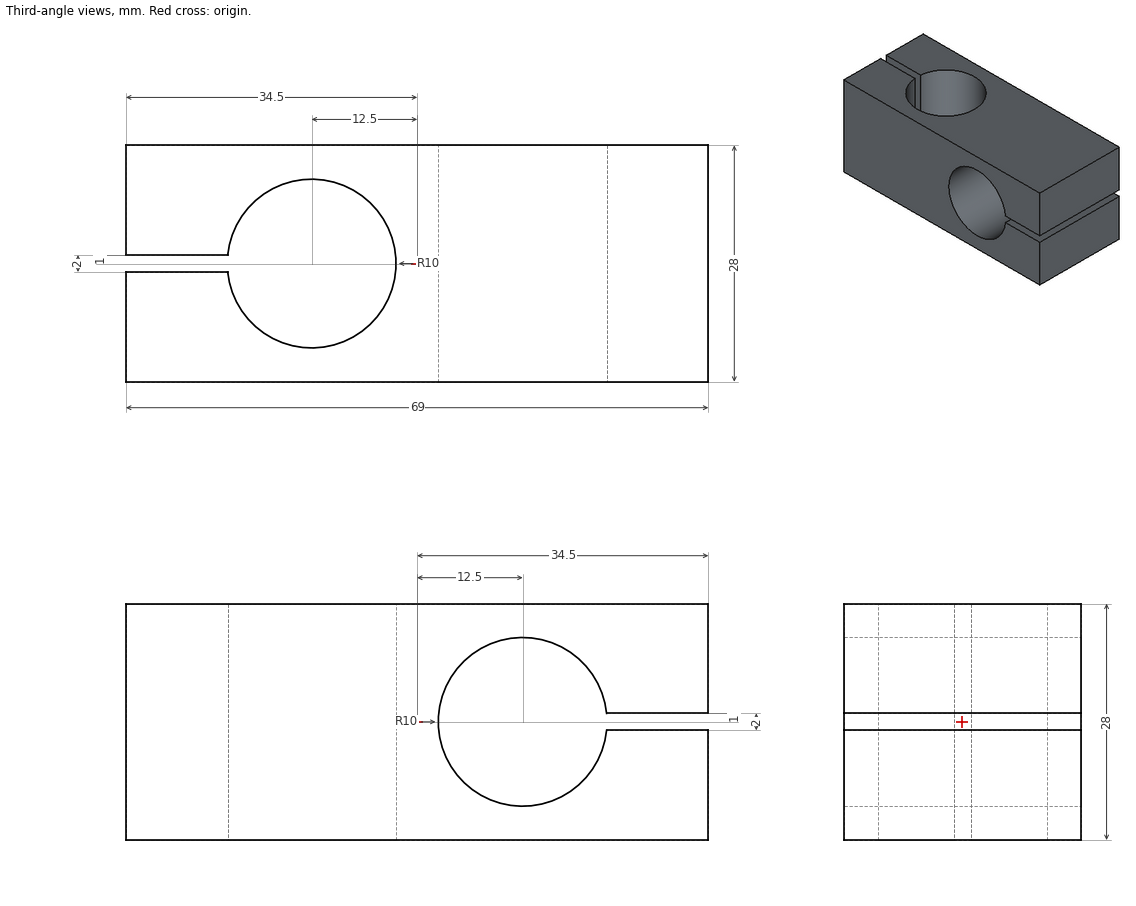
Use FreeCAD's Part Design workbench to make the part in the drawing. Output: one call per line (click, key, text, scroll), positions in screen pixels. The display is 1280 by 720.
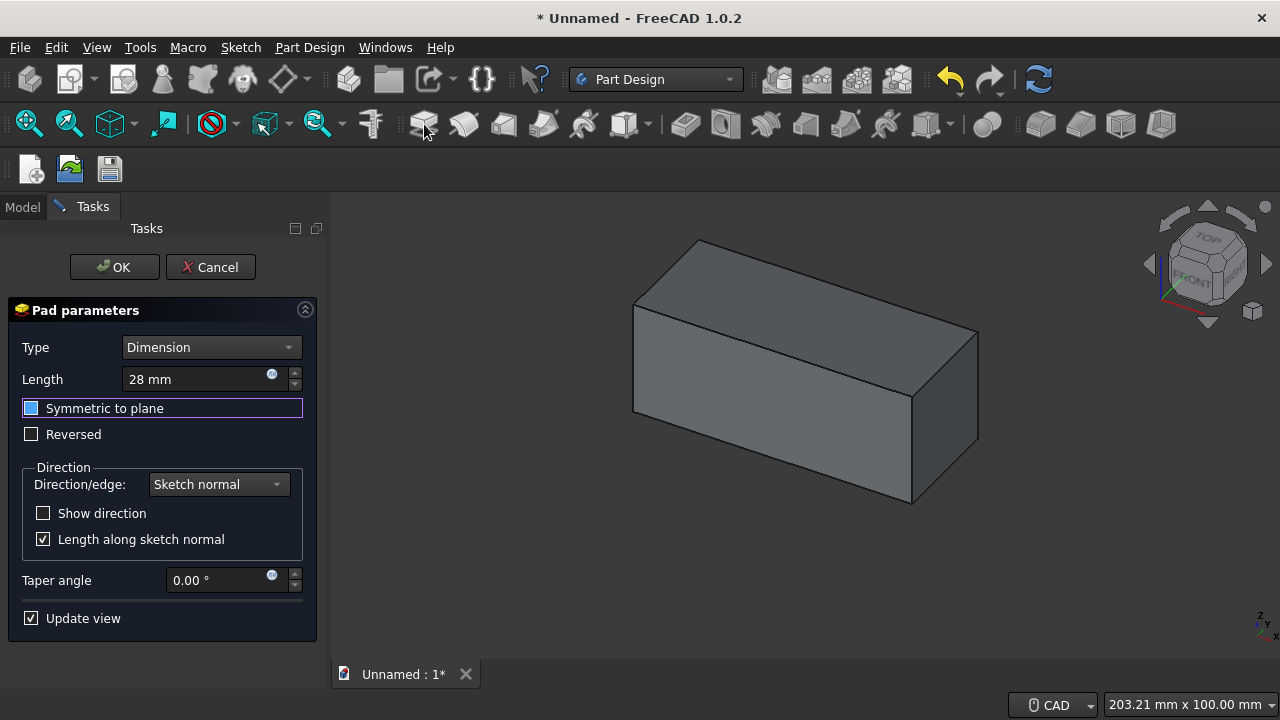
click(30, 408)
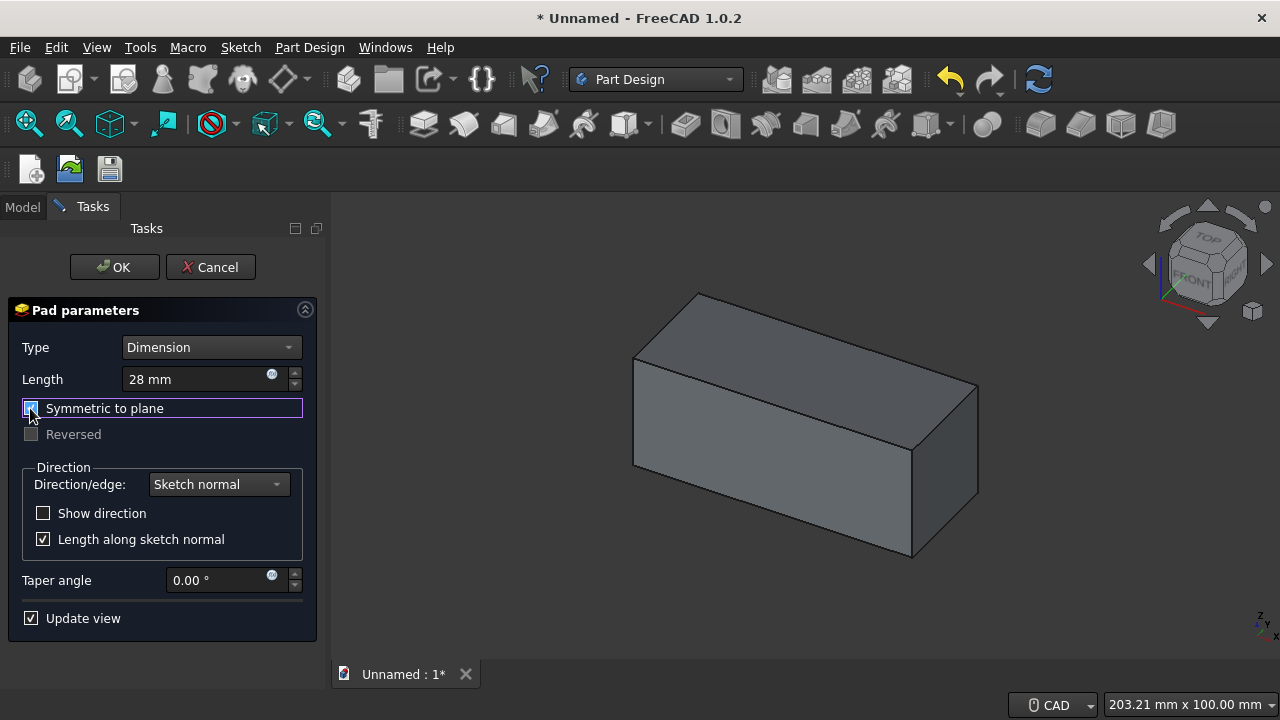
click(115, 267)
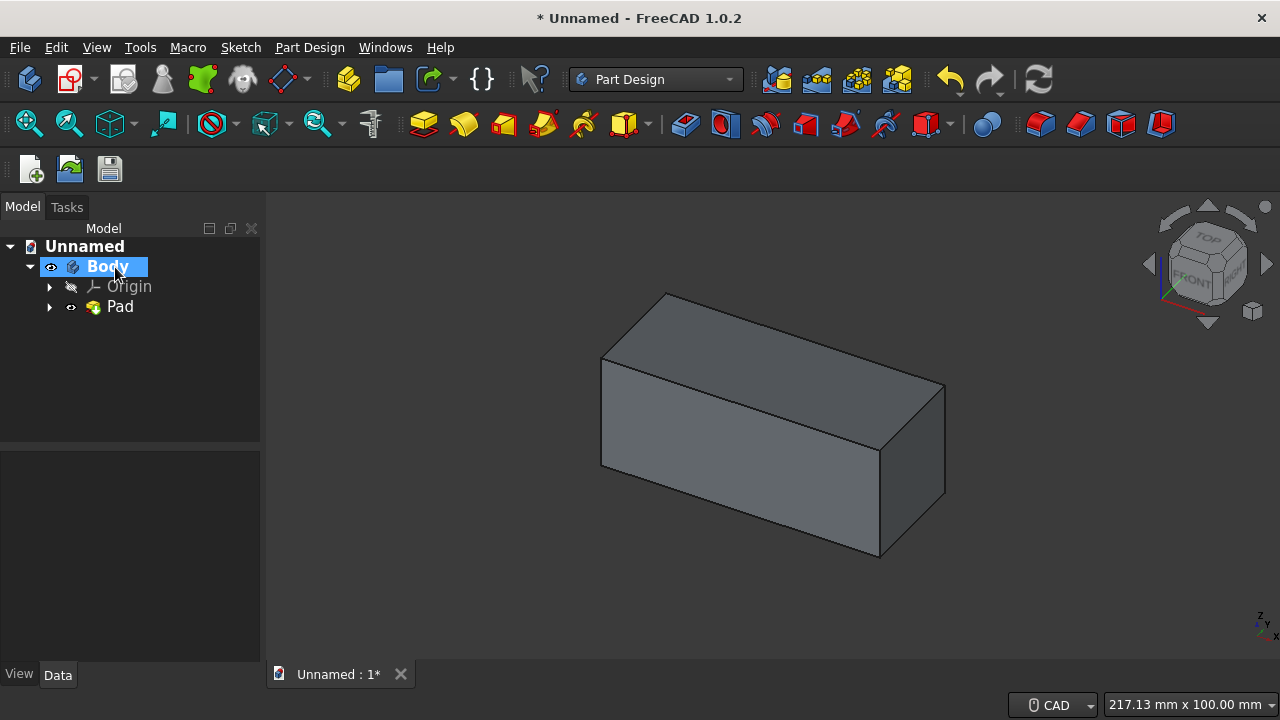
click(853, 397)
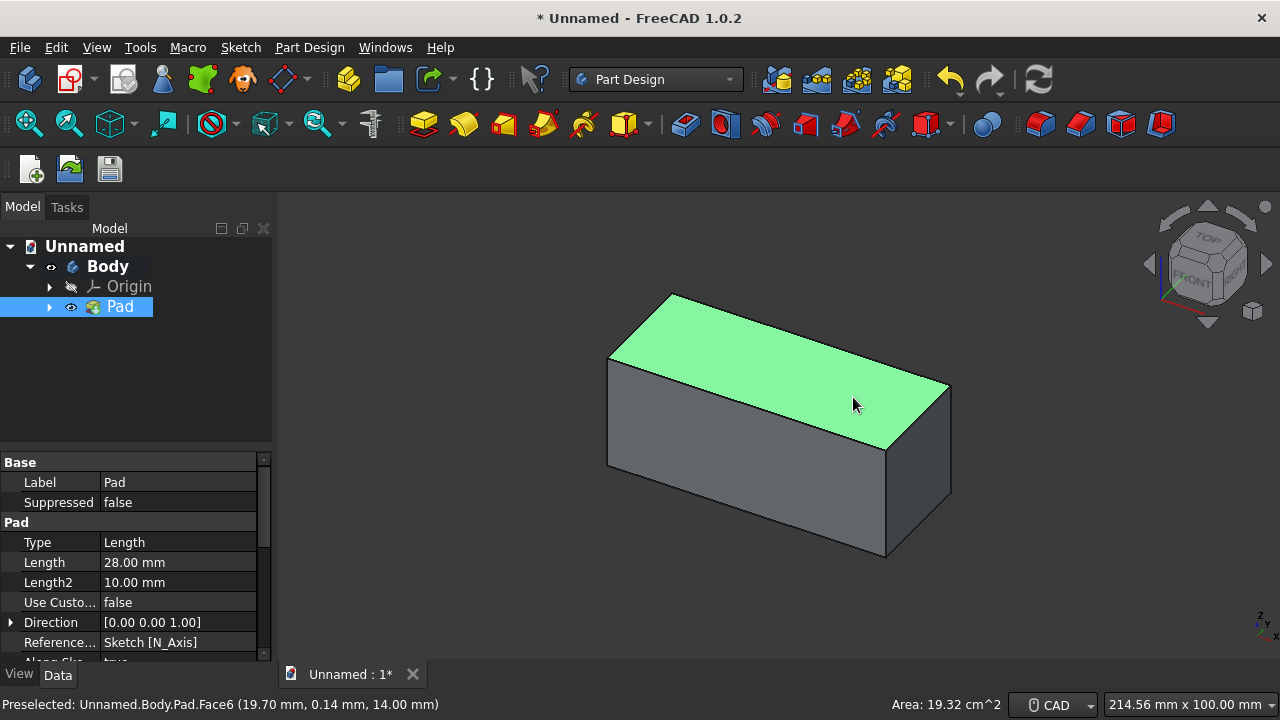
click(70, 80)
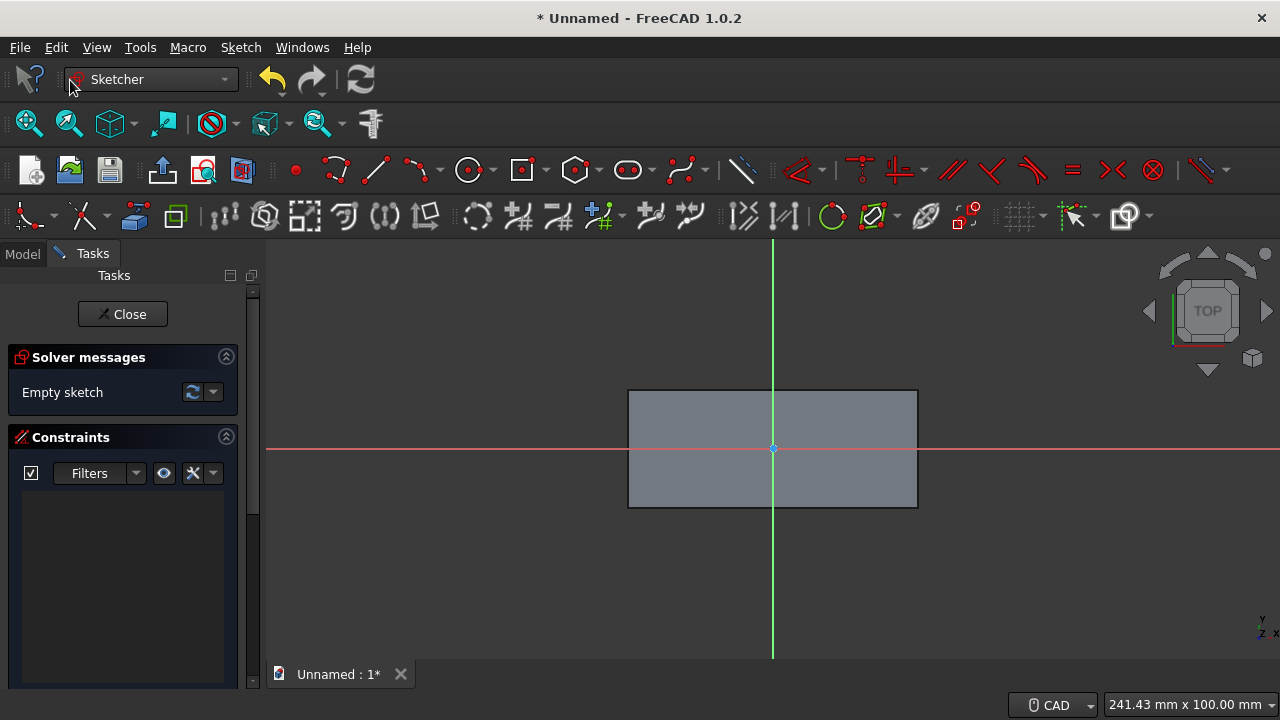
scroll(699, 449, up, 7)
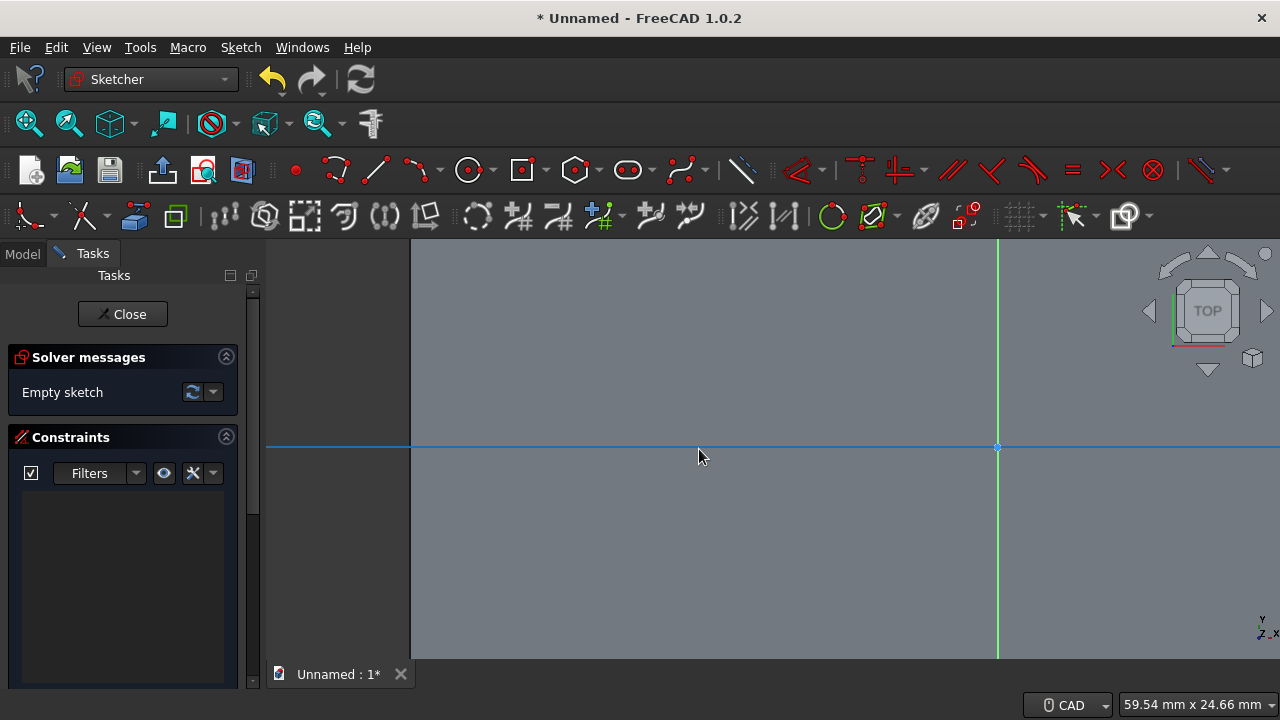
click(336, 170)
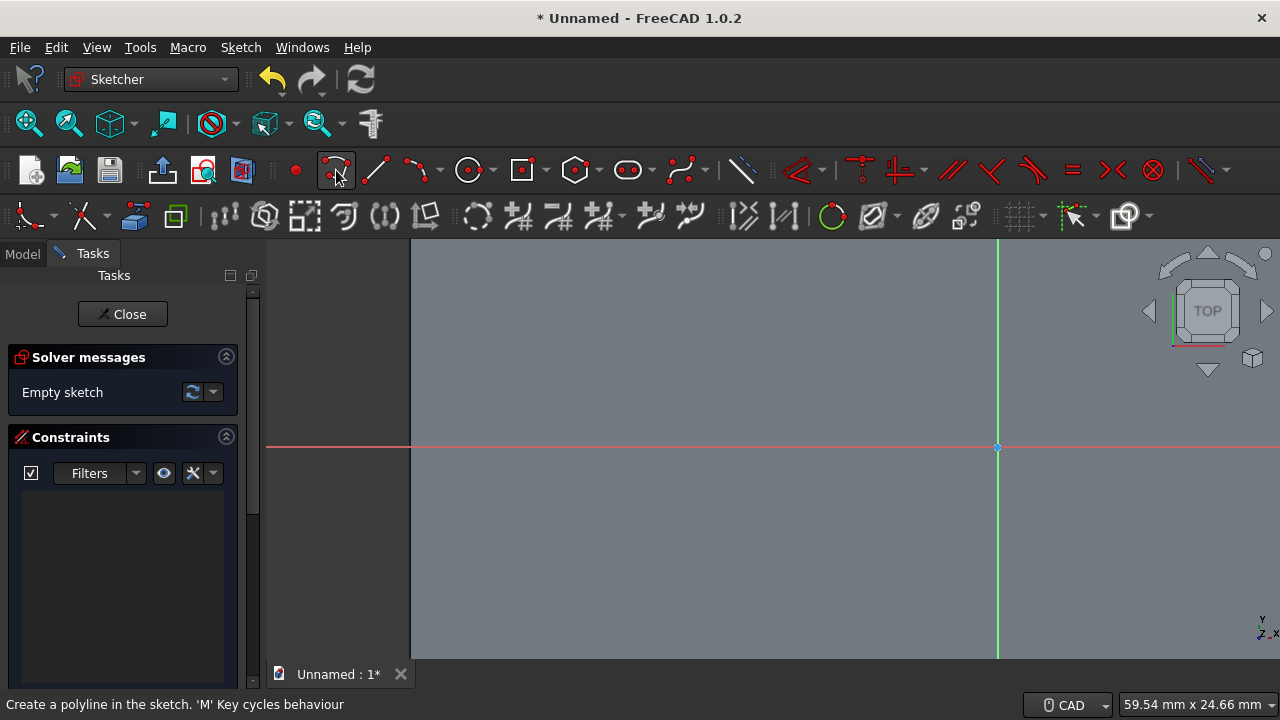
click(615, 430)
click(410, 430)
click(410, 465)
click(615, 465)
right_click(615, 465)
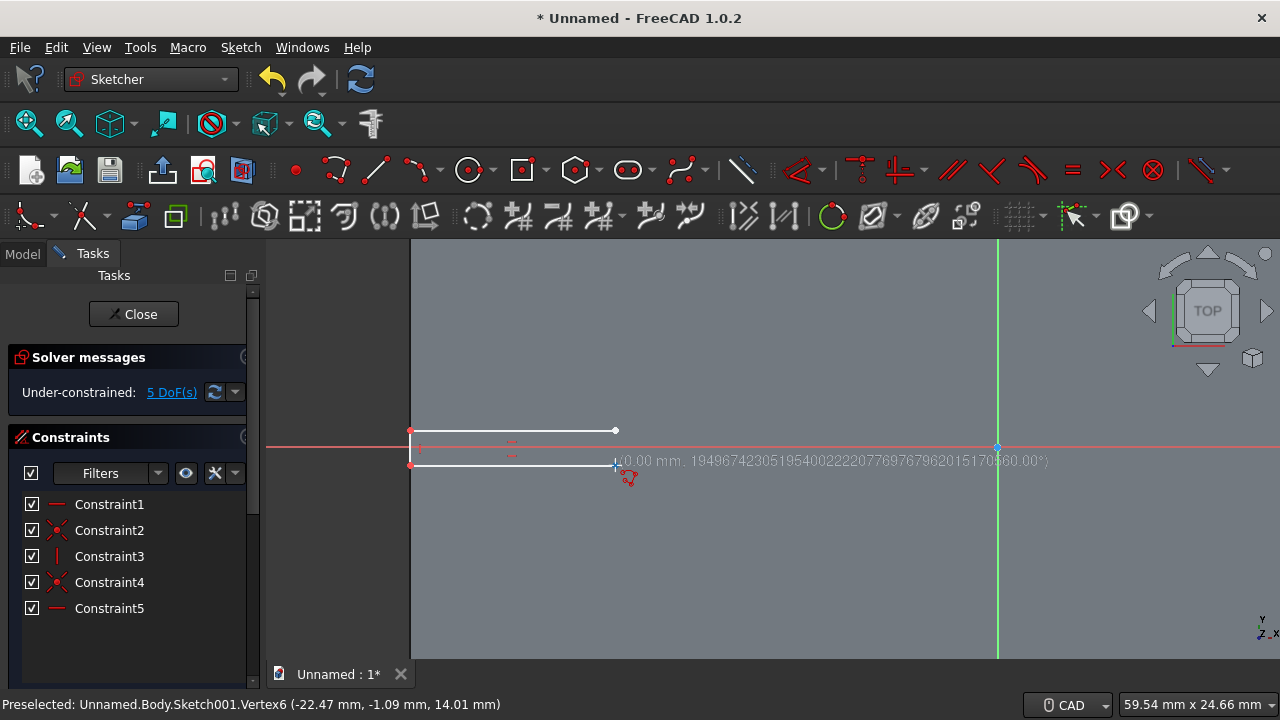
key(g)
key(3)
key(a)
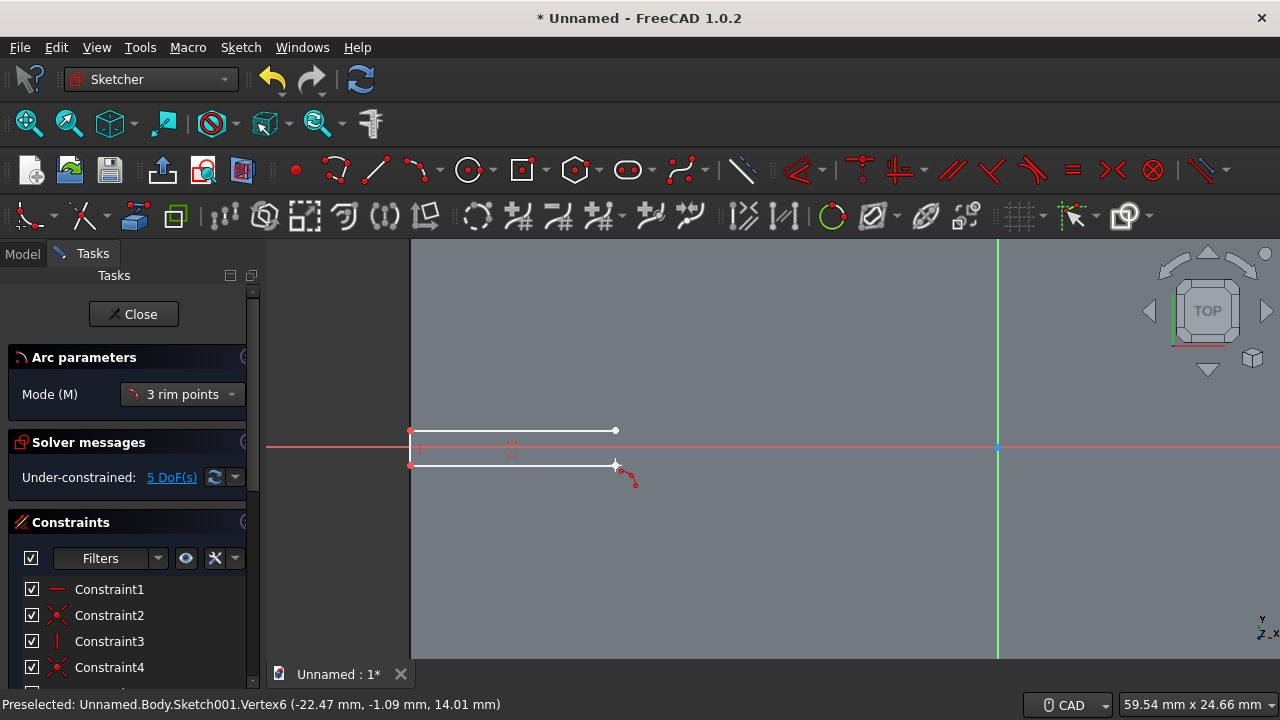
click(615, 466)
click(615, 431)
click(925, 545)
key(Escape)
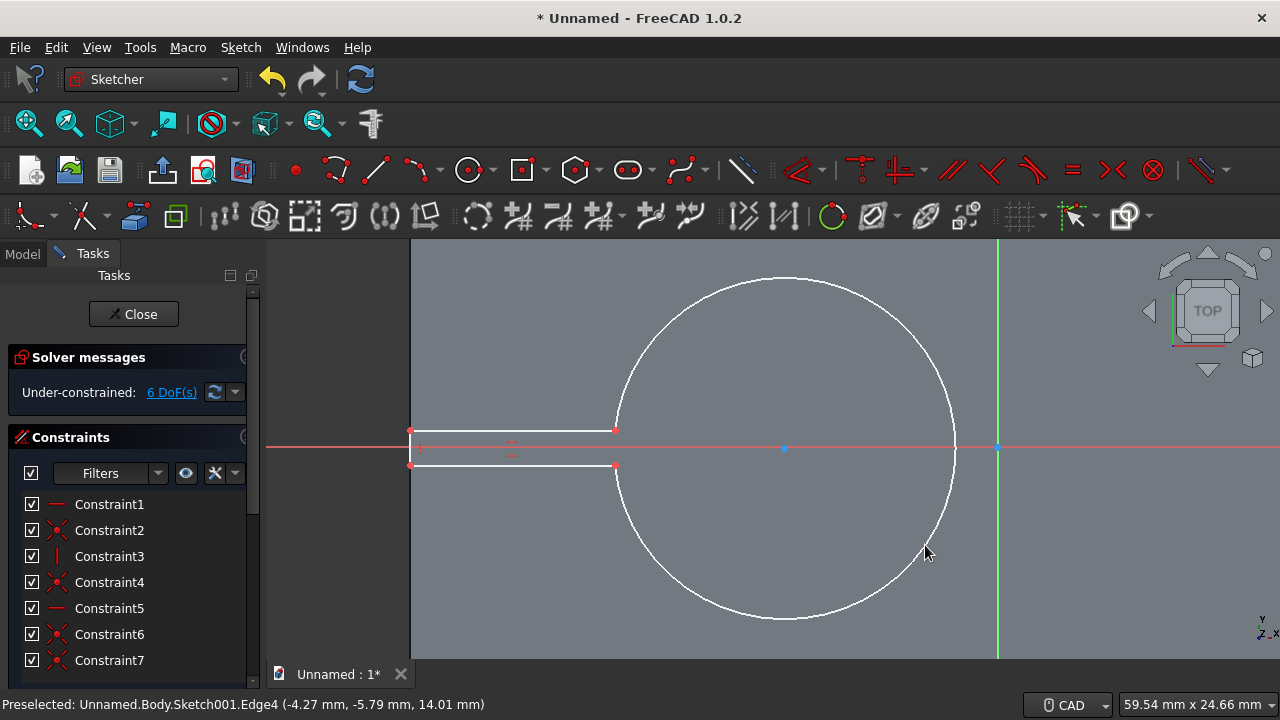
click(785, 449)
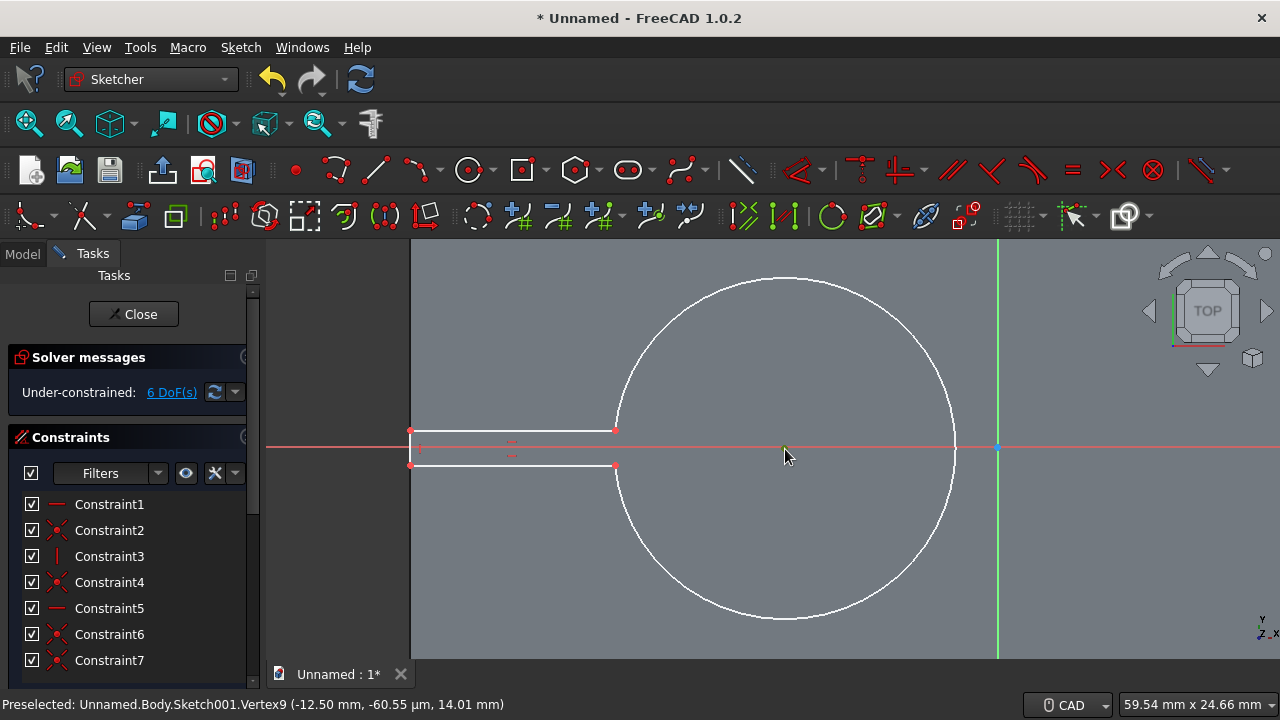
click(353, 447)